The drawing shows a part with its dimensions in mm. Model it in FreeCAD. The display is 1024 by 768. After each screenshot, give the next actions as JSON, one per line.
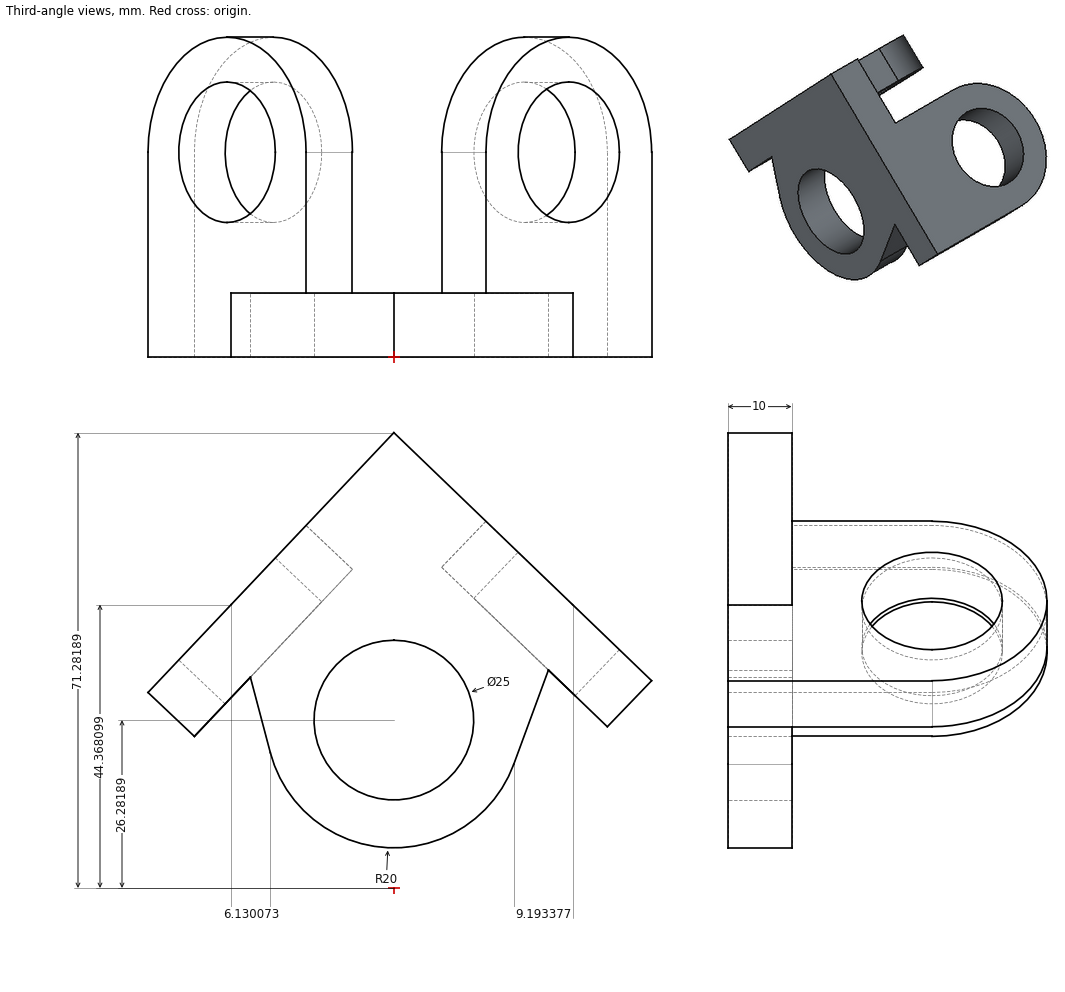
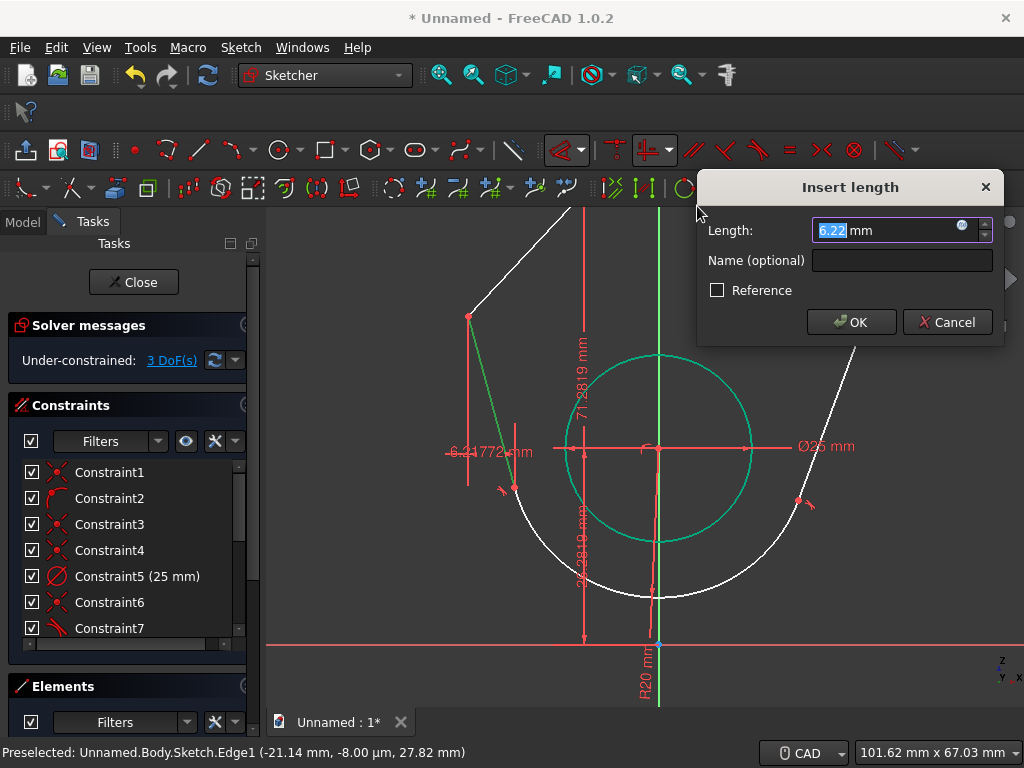
{"action": "type", "text": "6.130073"}
{"action": "key", "text": "Return"}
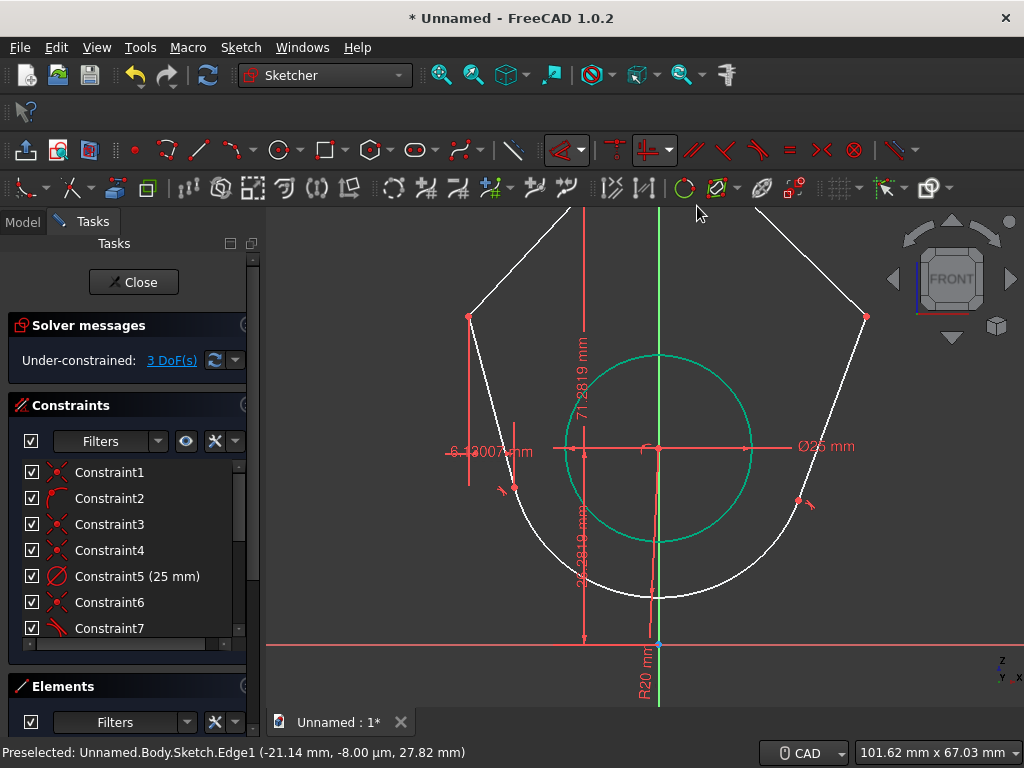
{"action": "left_click", "coordinate": [846, 371]}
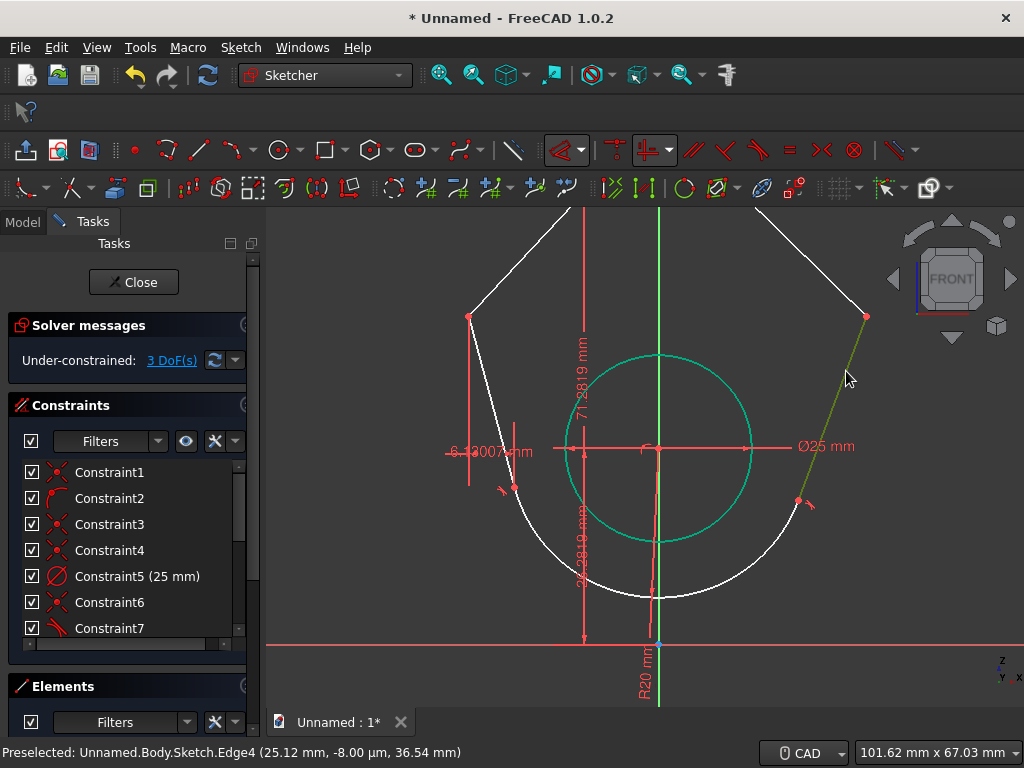
{"action": "key", "text": "l"}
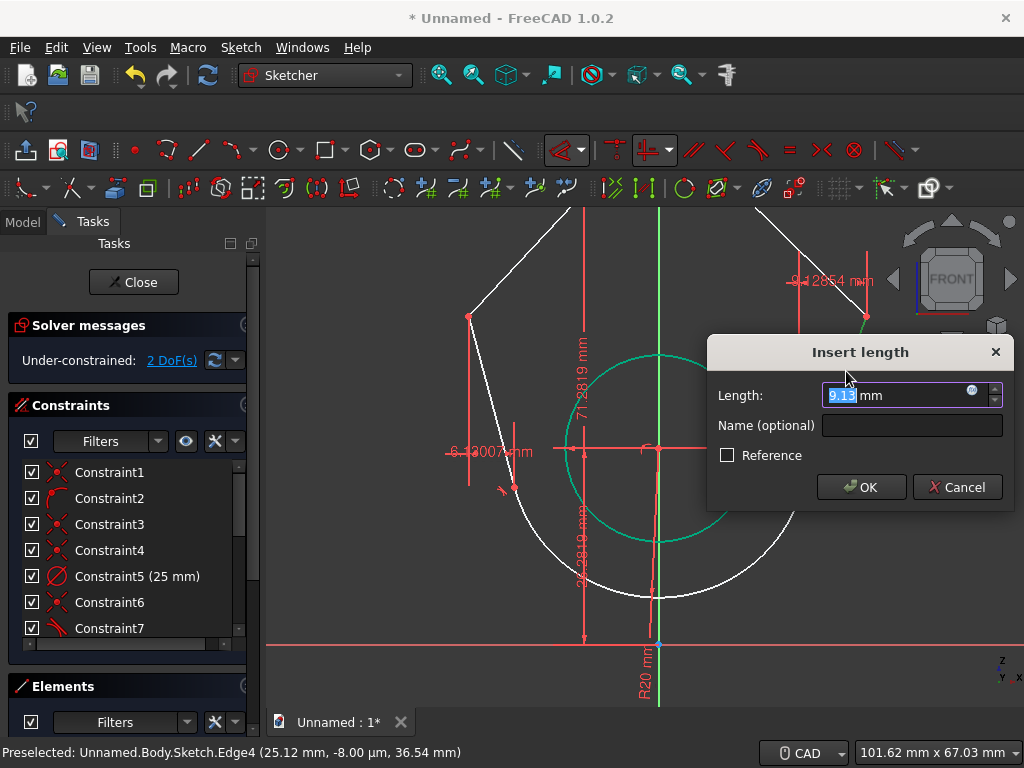
{"action": "type", "text": "9.193377"}
{"action": "key", "text": "Return"}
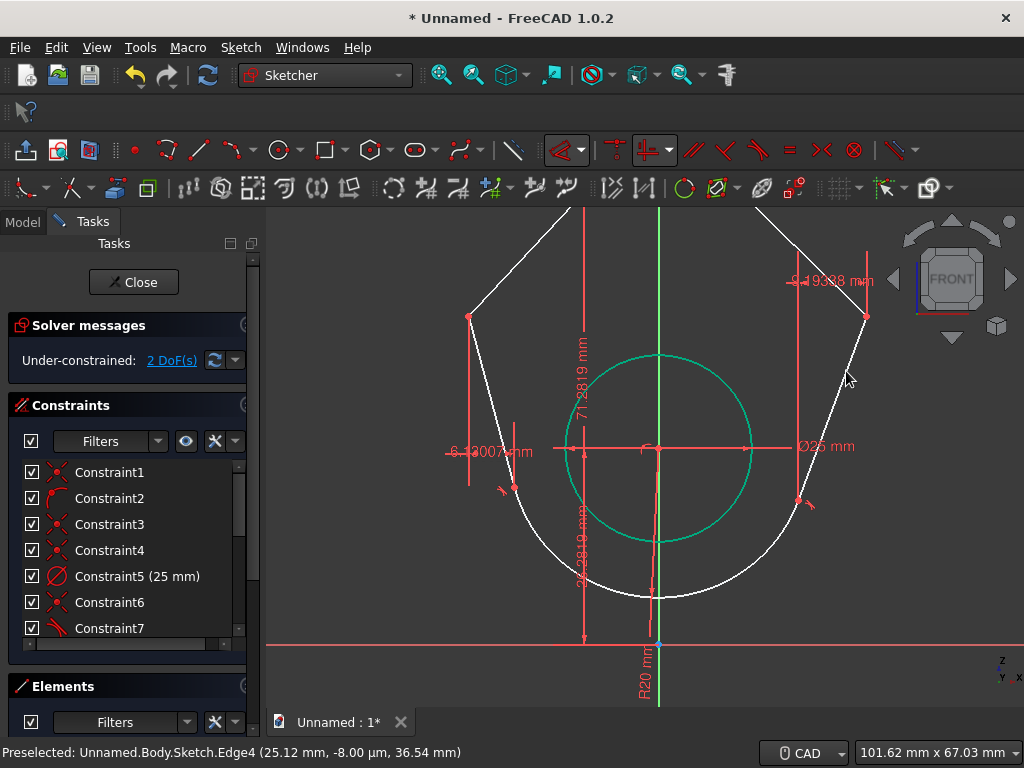
{"action": "left_click", "coordinate": [469, 316]}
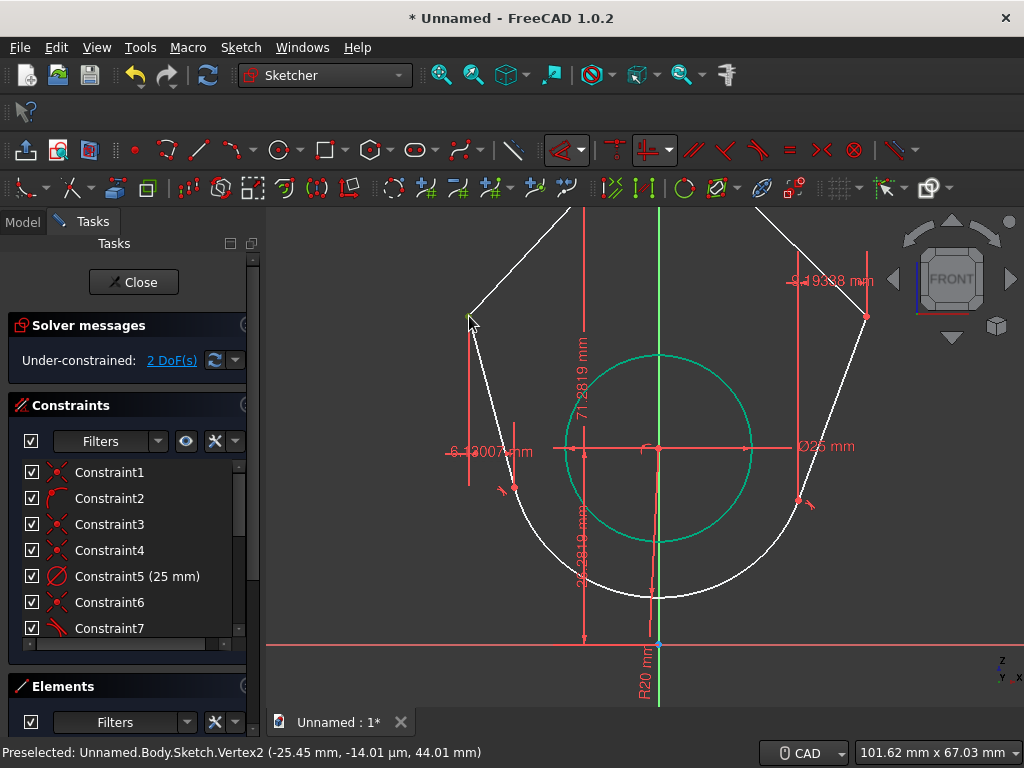
{"action": "key", "text": "i"}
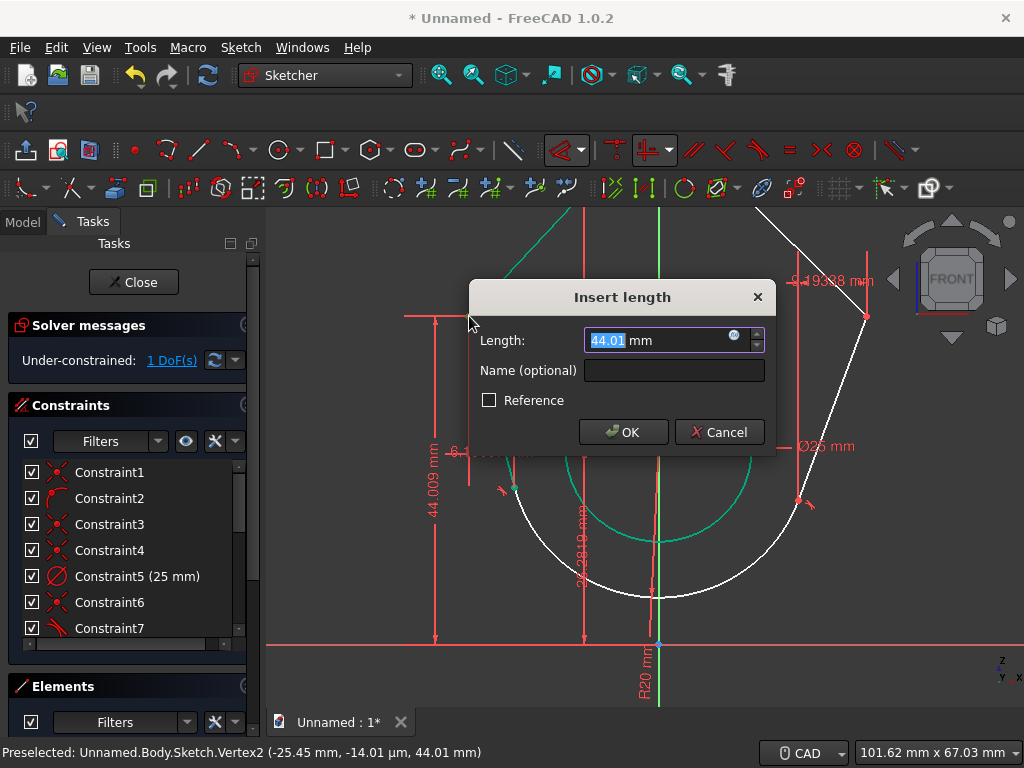
{"action": "type", "text": "44.368099"}
{"action": "key", "text": "Return"}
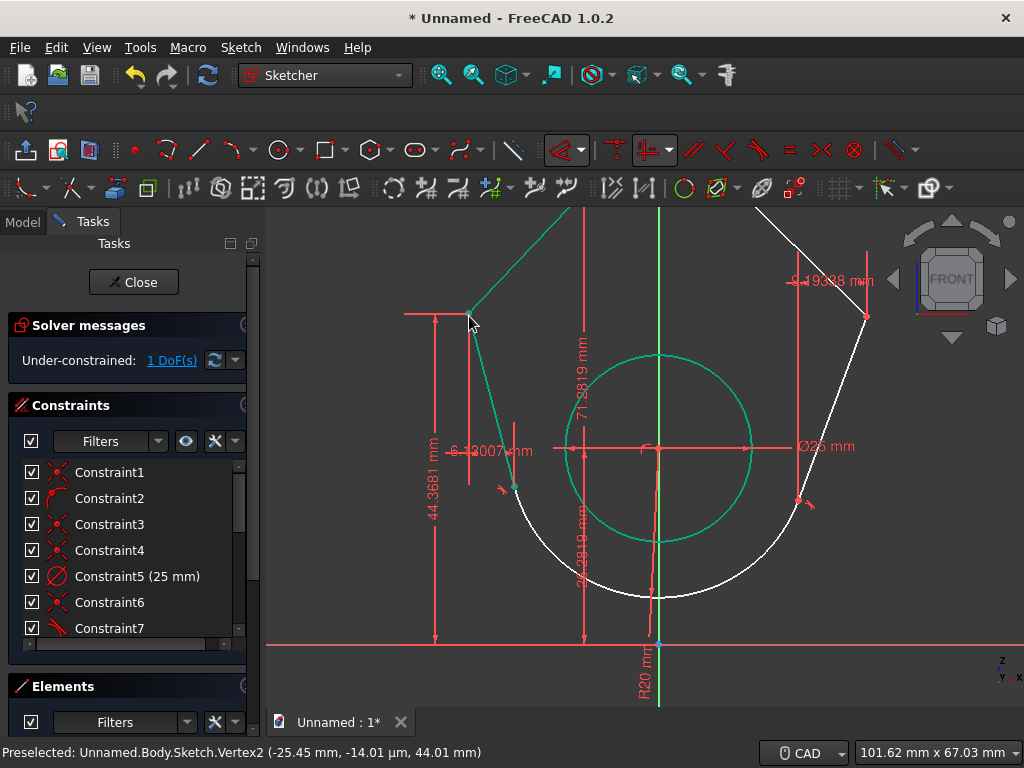
{"action": "scroll", "coordinate": [465, 552], "scroll_direction": "down", "scroll_amount": 3}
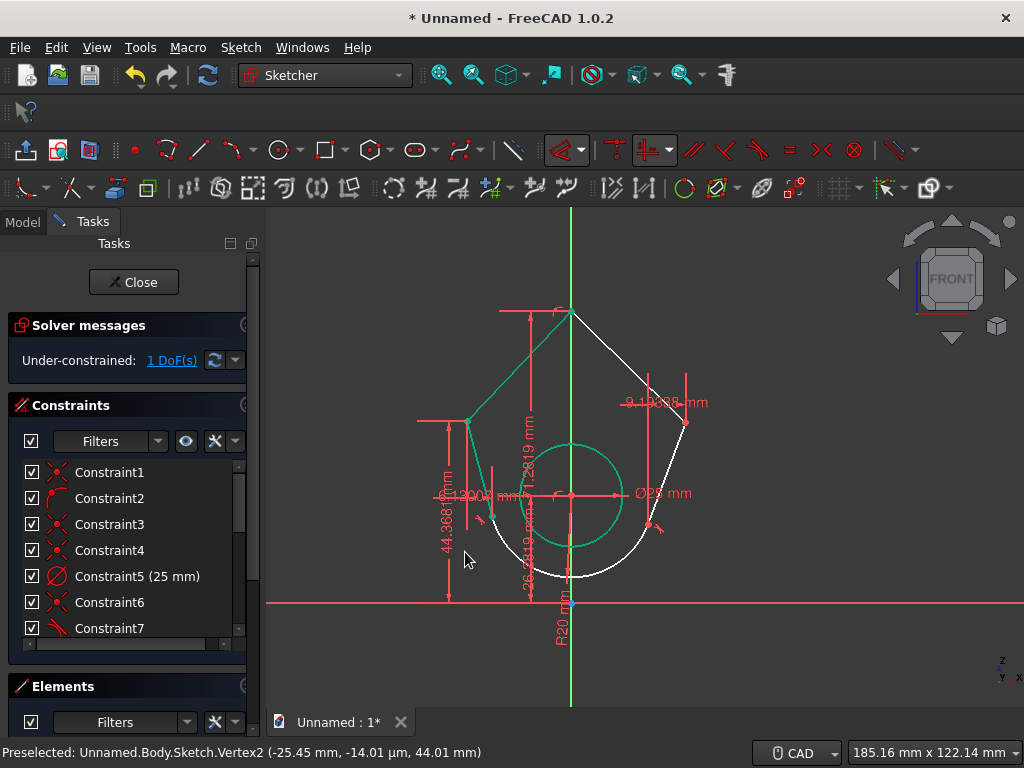
{"action": "left_click", "coordinate": [686, 423]}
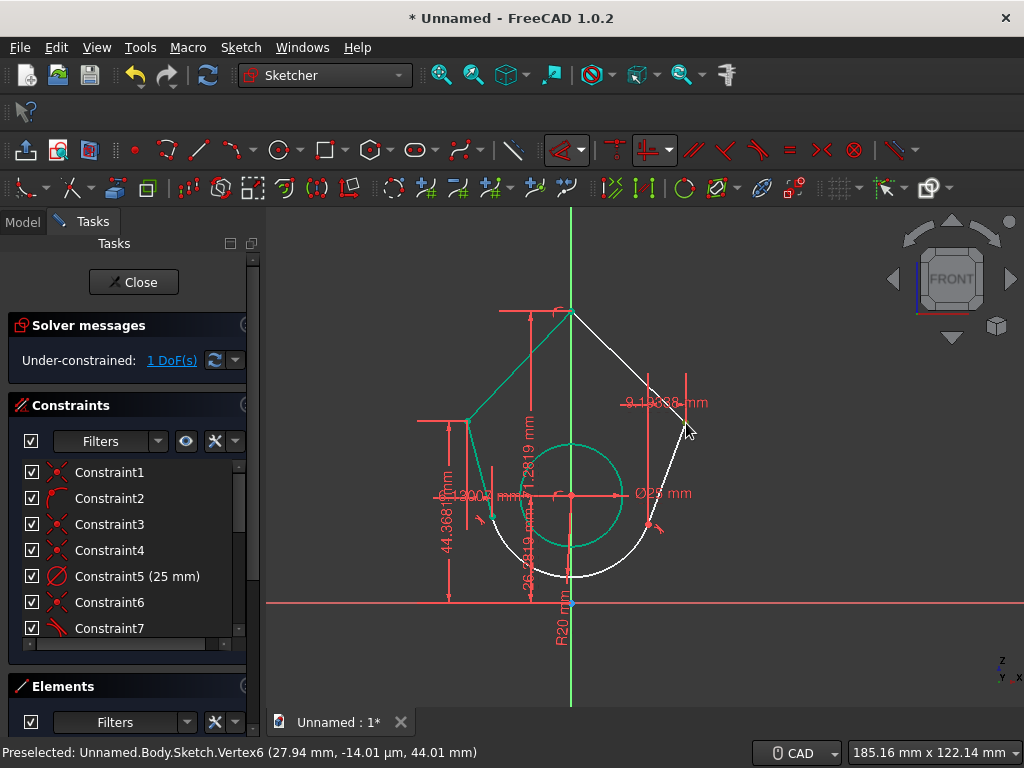
{"action": "key", "text": "i"}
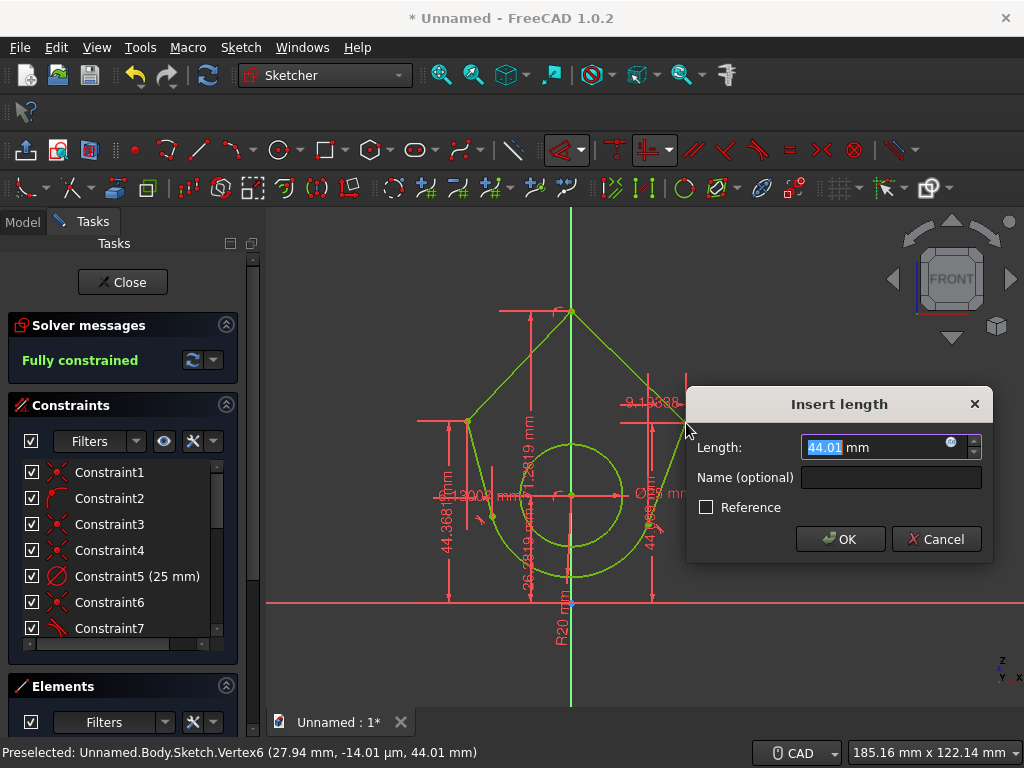
{"action": "type", "text": "44.368099"}
{"action": "key", "text": "Return"}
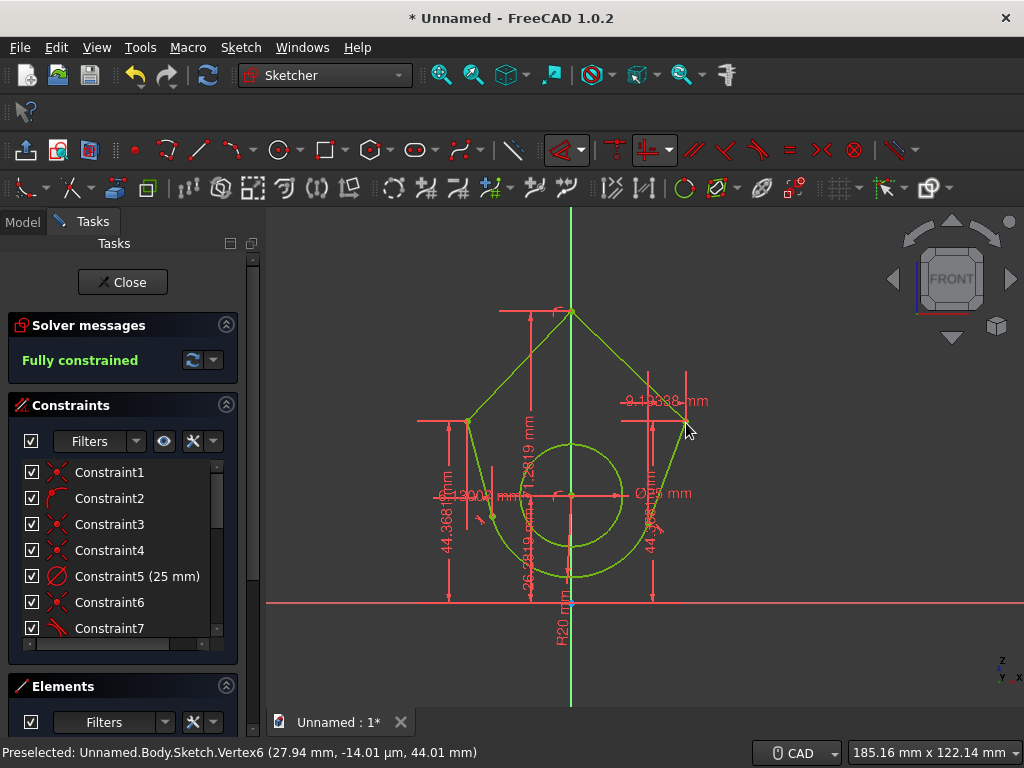
{"action": "left_click", "coordinate": [123, 282]}